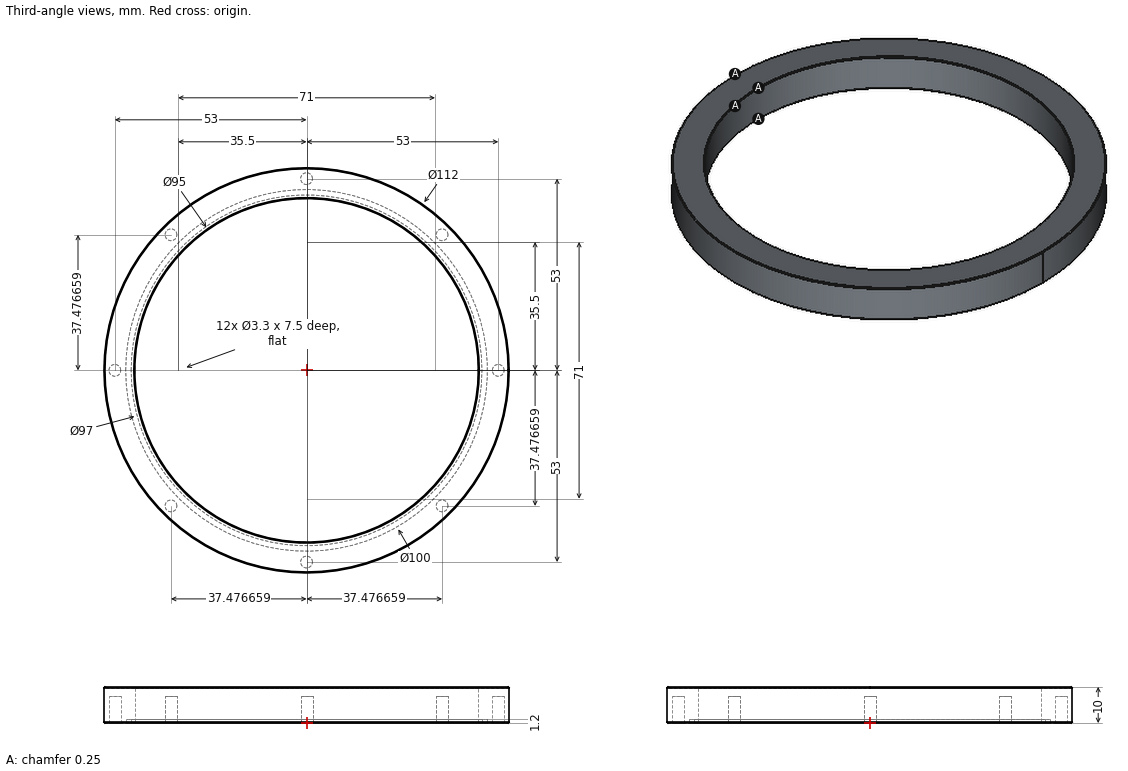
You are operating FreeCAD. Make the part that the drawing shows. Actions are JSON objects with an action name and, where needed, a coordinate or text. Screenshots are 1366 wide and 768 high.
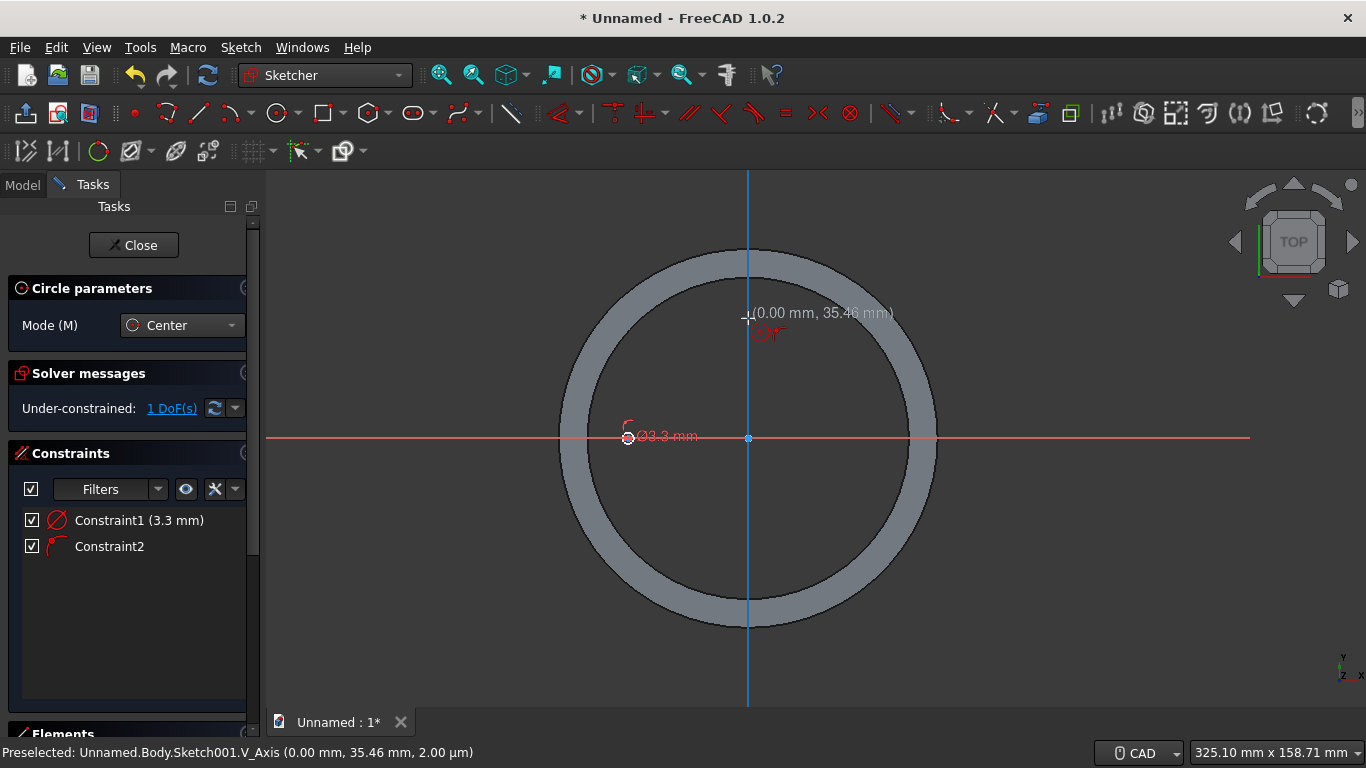
{"action": "left_click", "coordinate": [748, 318]}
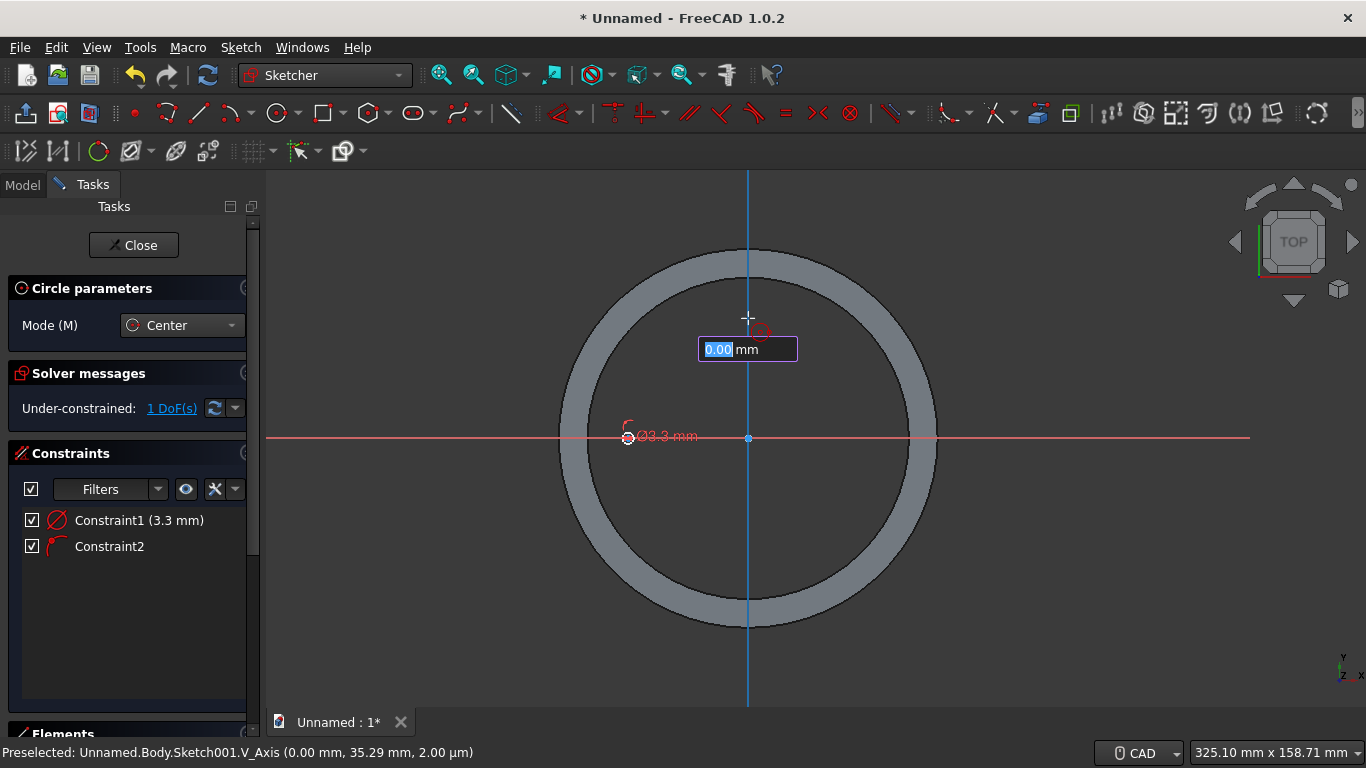
{"action": "scroll", "coordinate": [753, 316], "scroll_direction": "up", "scroll_amount": 6}
{"action": "mouse_move", "coordinate": [753, 317]}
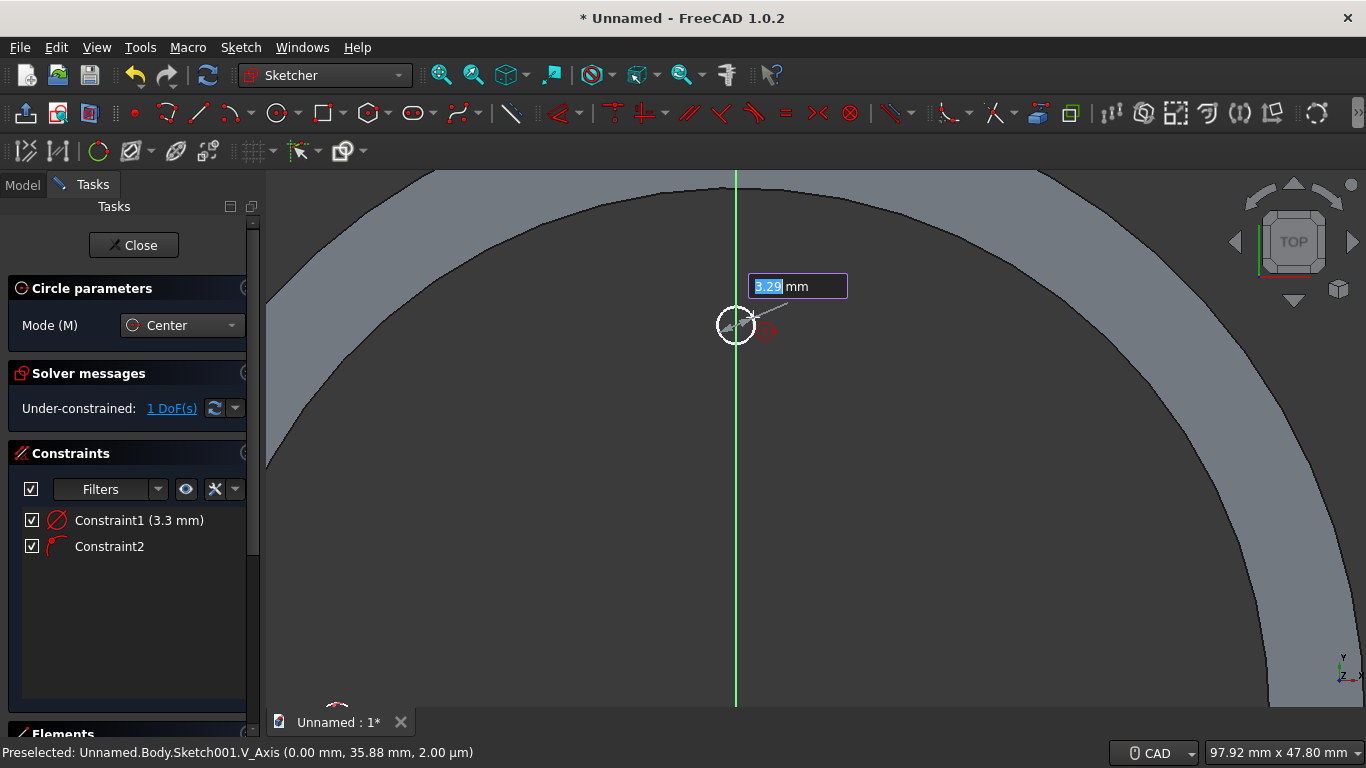
{"action": "type", "text": "3.3"}
{"action": "key", "text": "Return"}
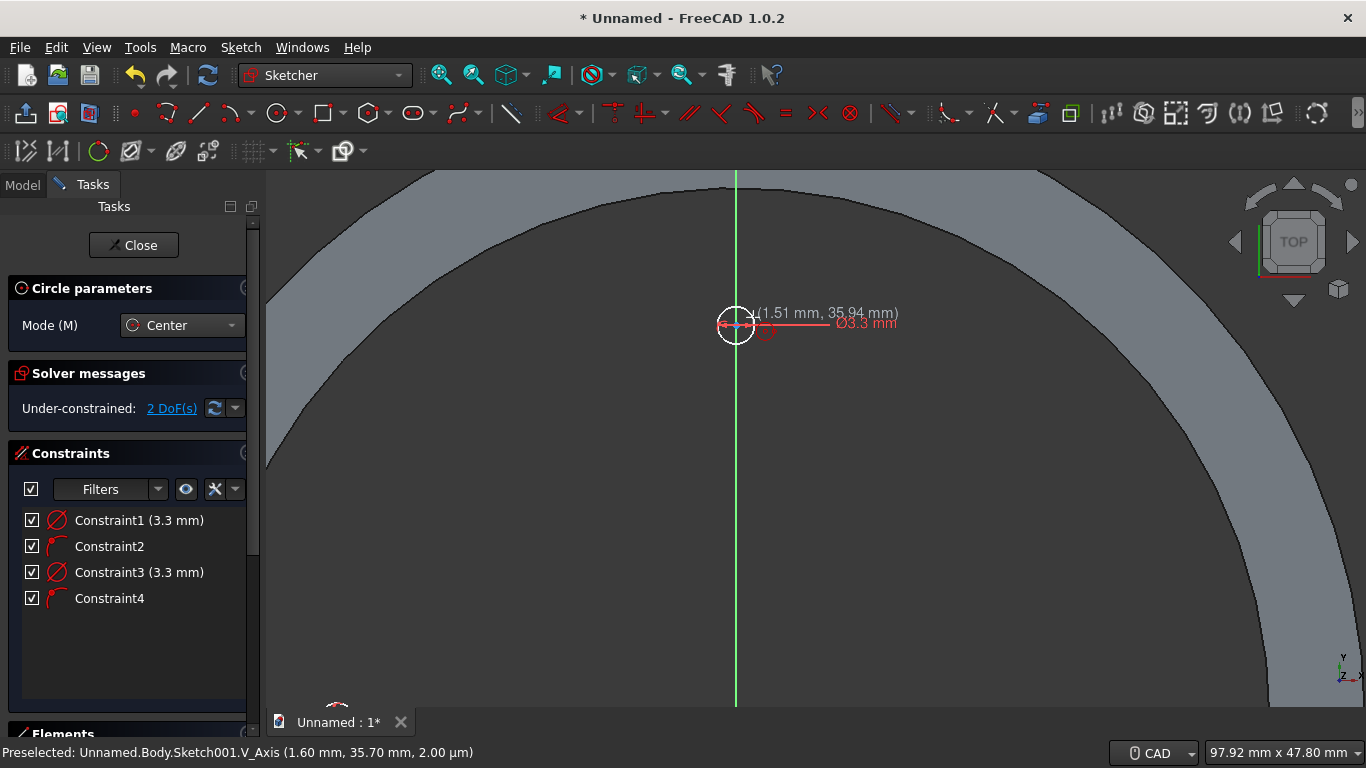
{"action": "scroll", "coordinate": [752, 316], "scroll_direction": "down", "scroll_amount": 6}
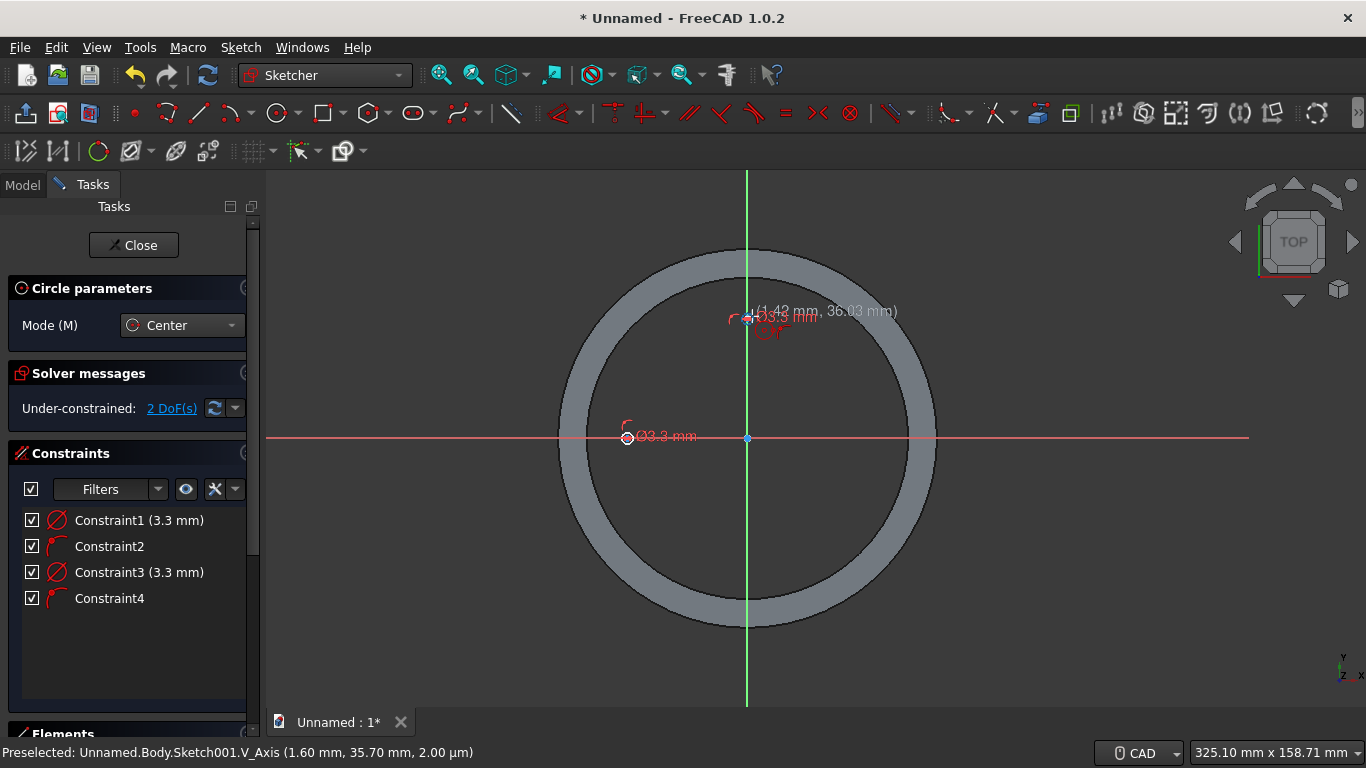
{"action": "scroll", "coordinate": [747, 559], "scroll_direction": "up", "scroll_amount": 8}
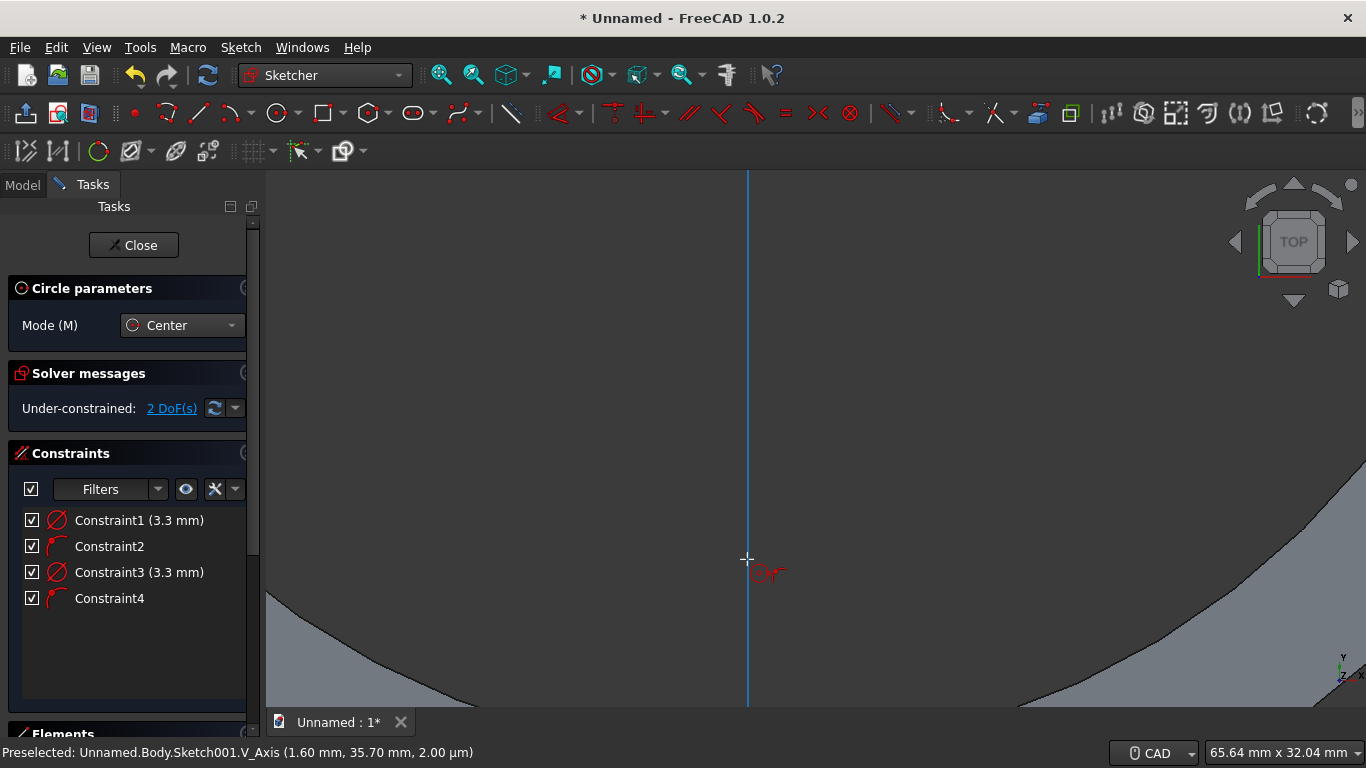
{"action": "scroll", "coordinate": [747, 560], "scroll_direction": "down", "scroll_amount": 8}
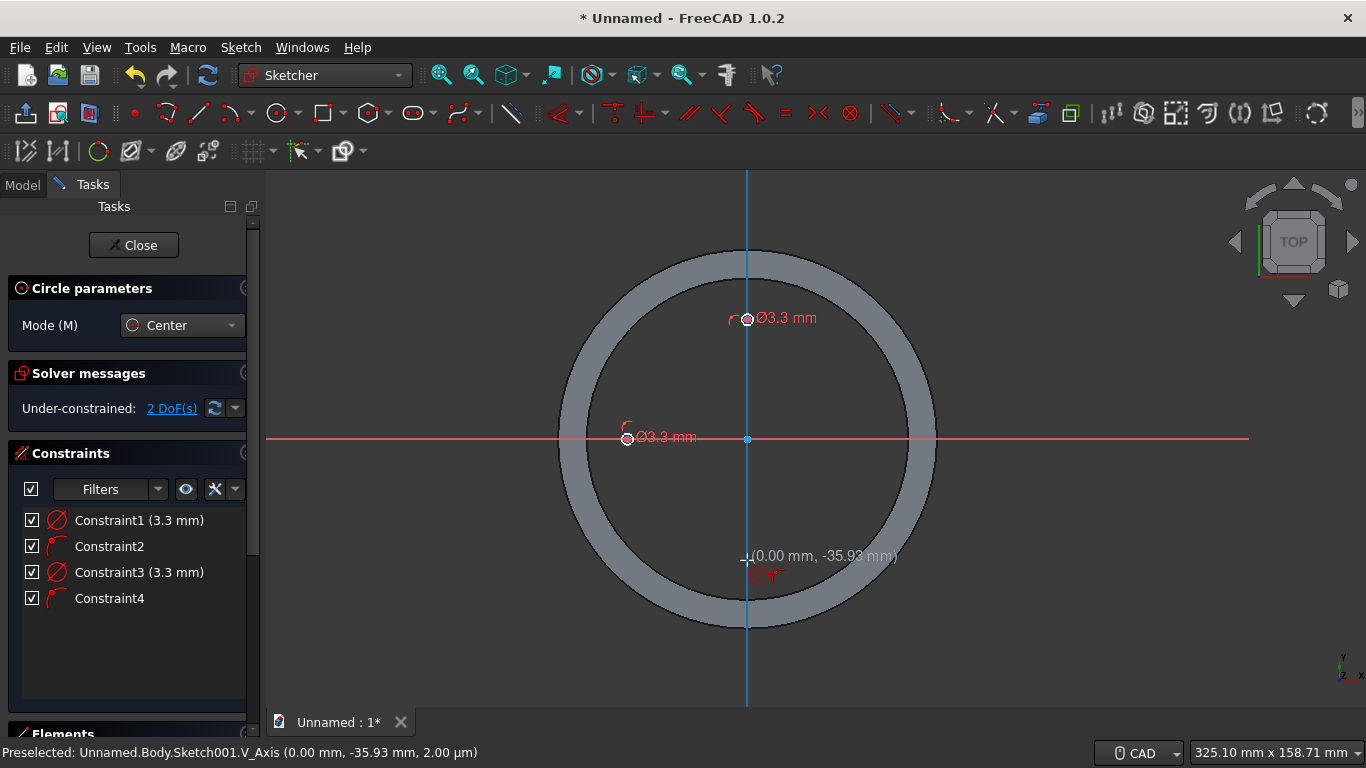
{"action": "left_click", "coordinate": [747, 559]}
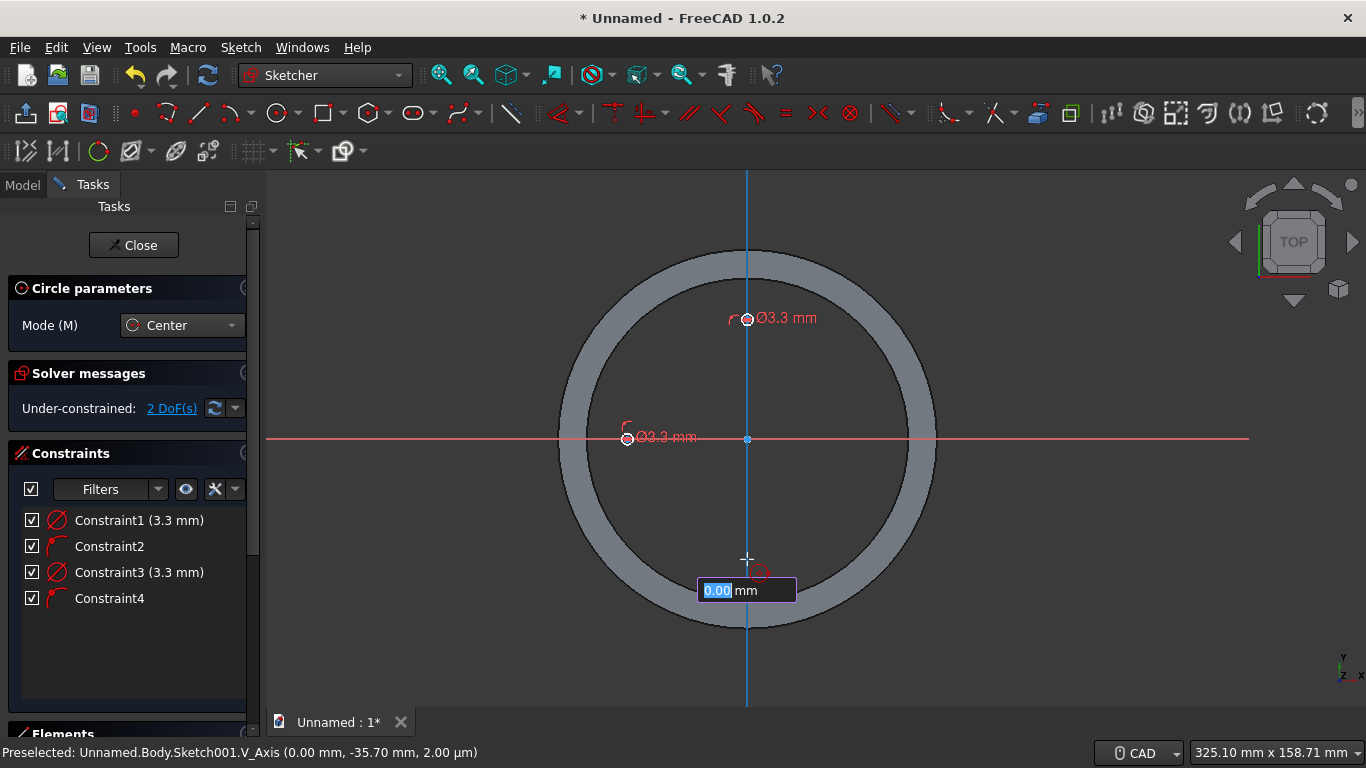
{"action": "scroll", "coordinate": [753, 557], "scroll_direction": "up", "scroll_amount": 6}
{"action": "mouse_move", "coordinate": [751, 557]}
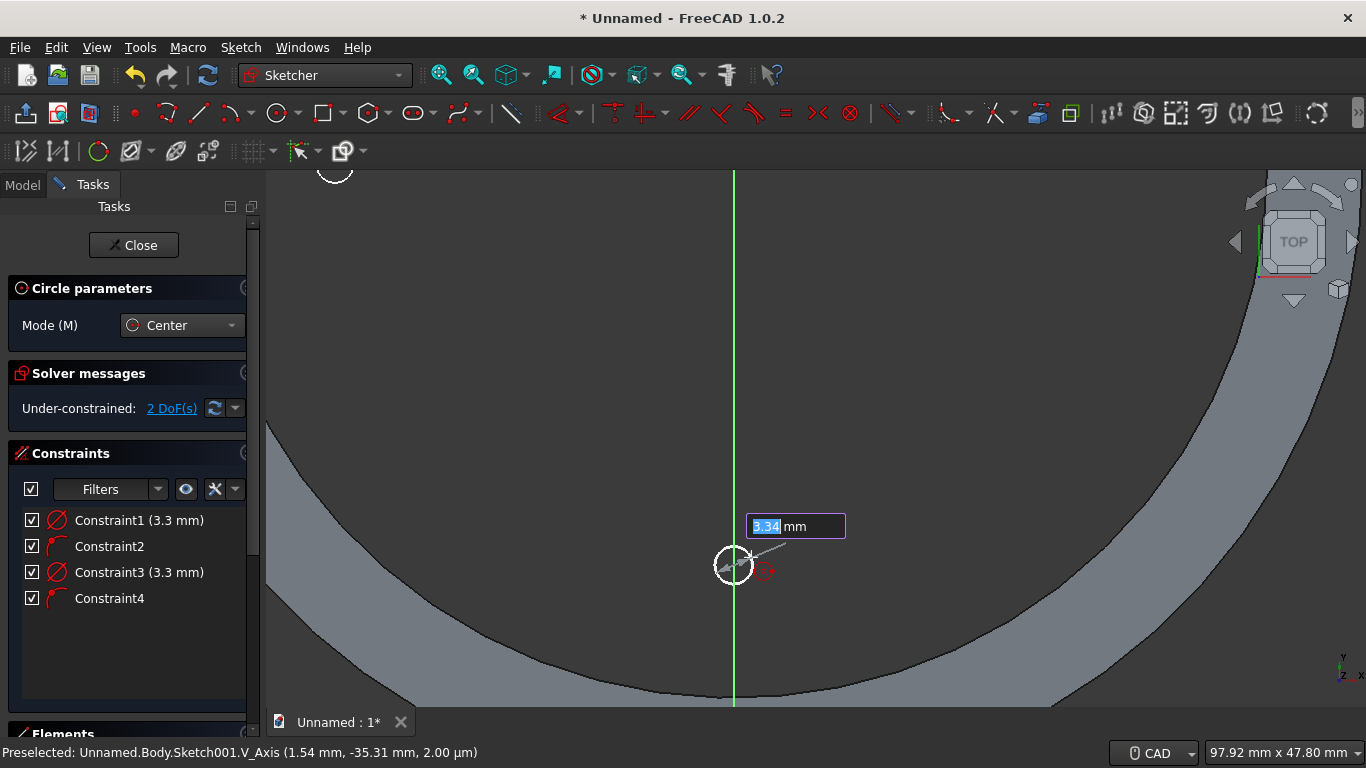
{"action": "type", "text": "3.3"}
{"action": "key", "text": "Return"}